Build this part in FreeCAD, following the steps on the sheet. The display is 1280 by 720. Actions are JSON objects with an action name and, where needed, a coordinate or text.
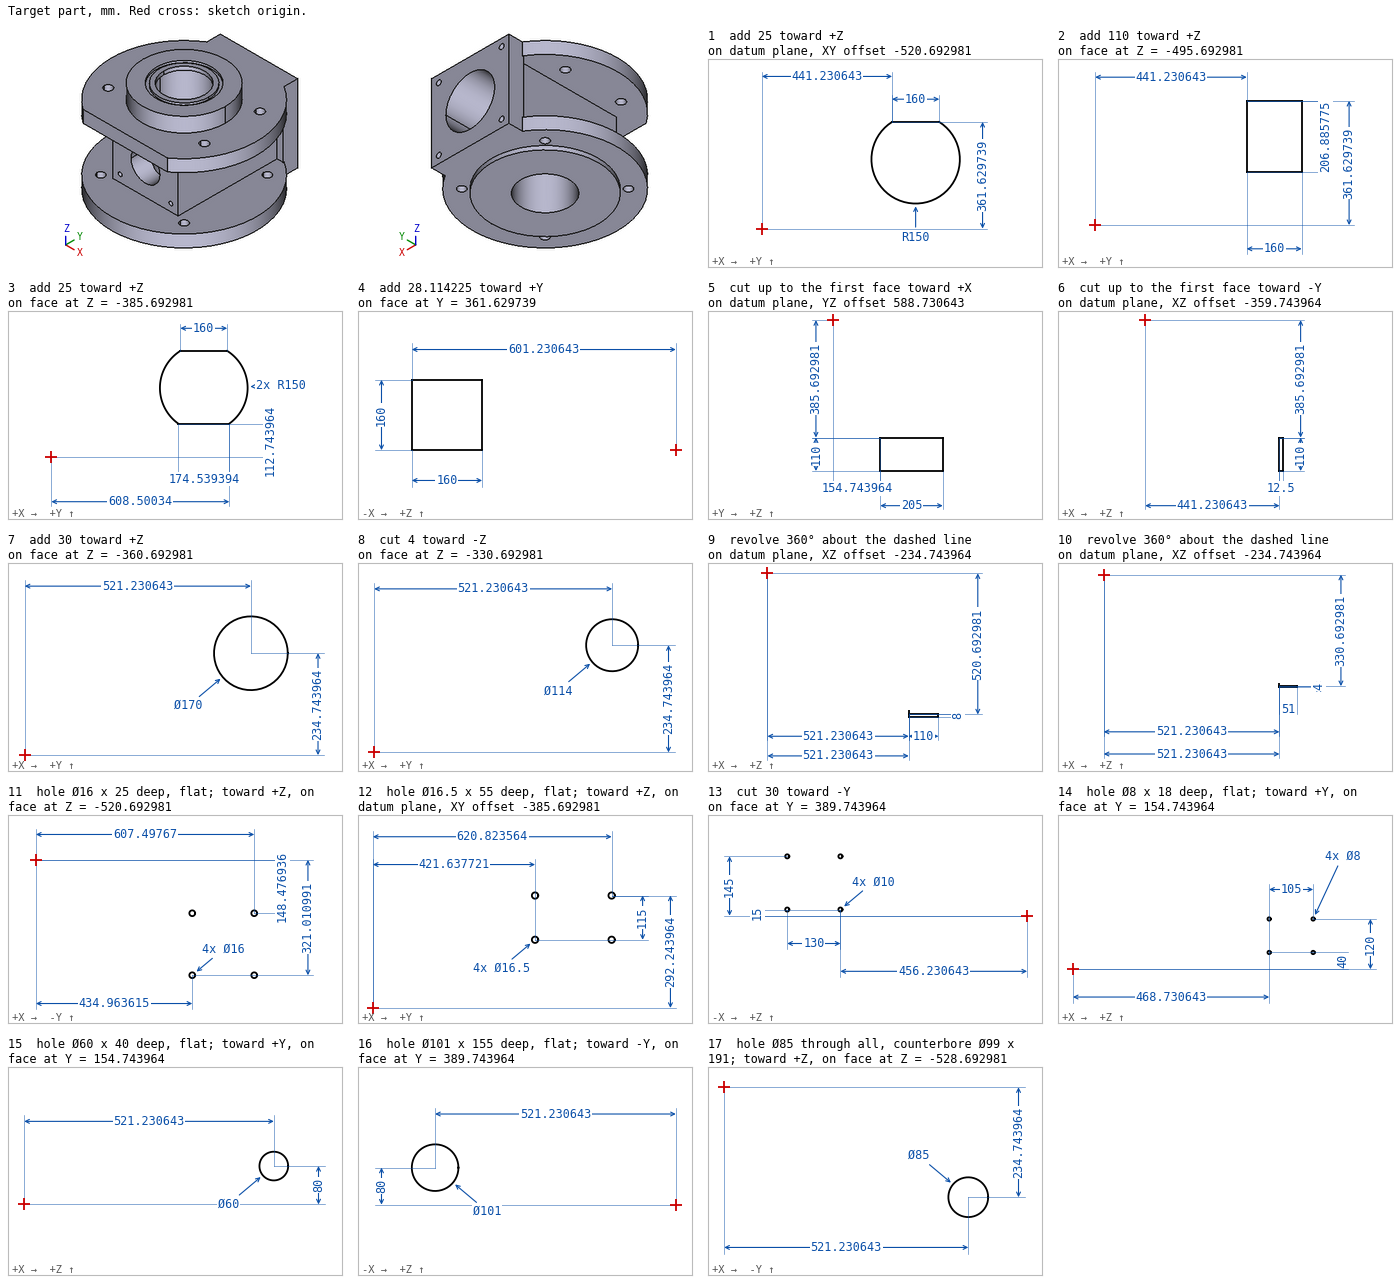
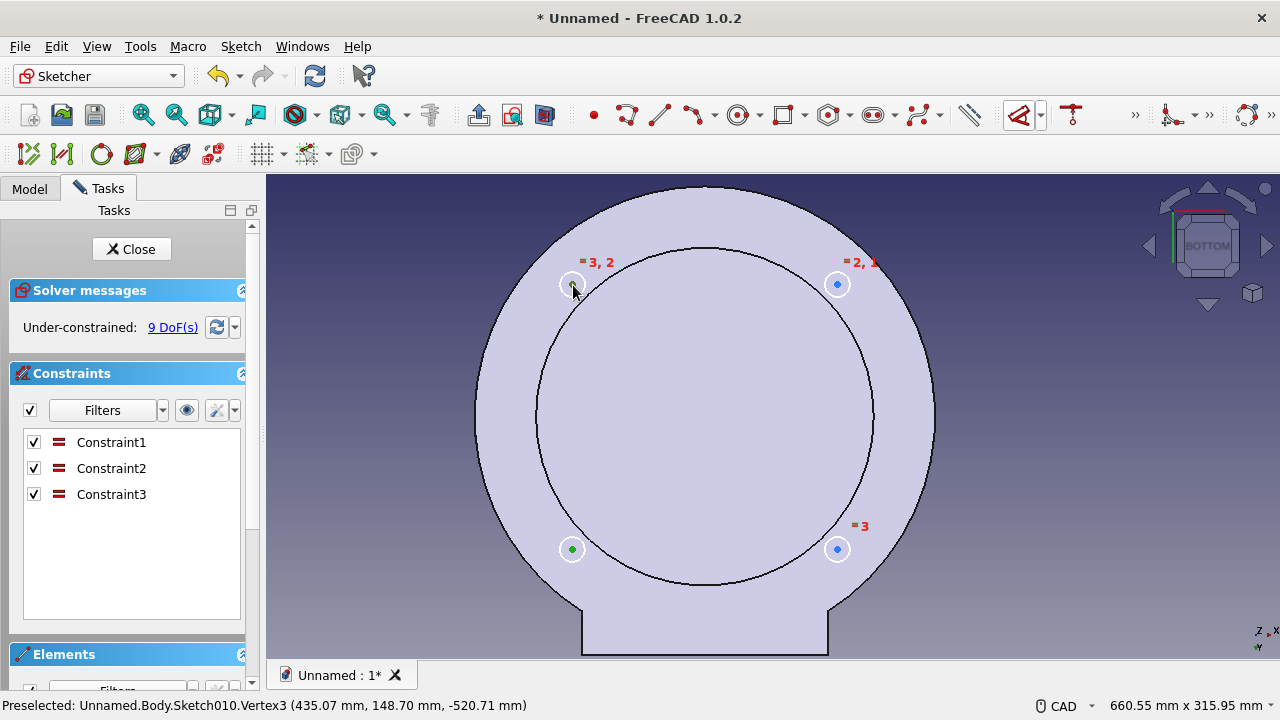
{"action": "key", "text": "v"}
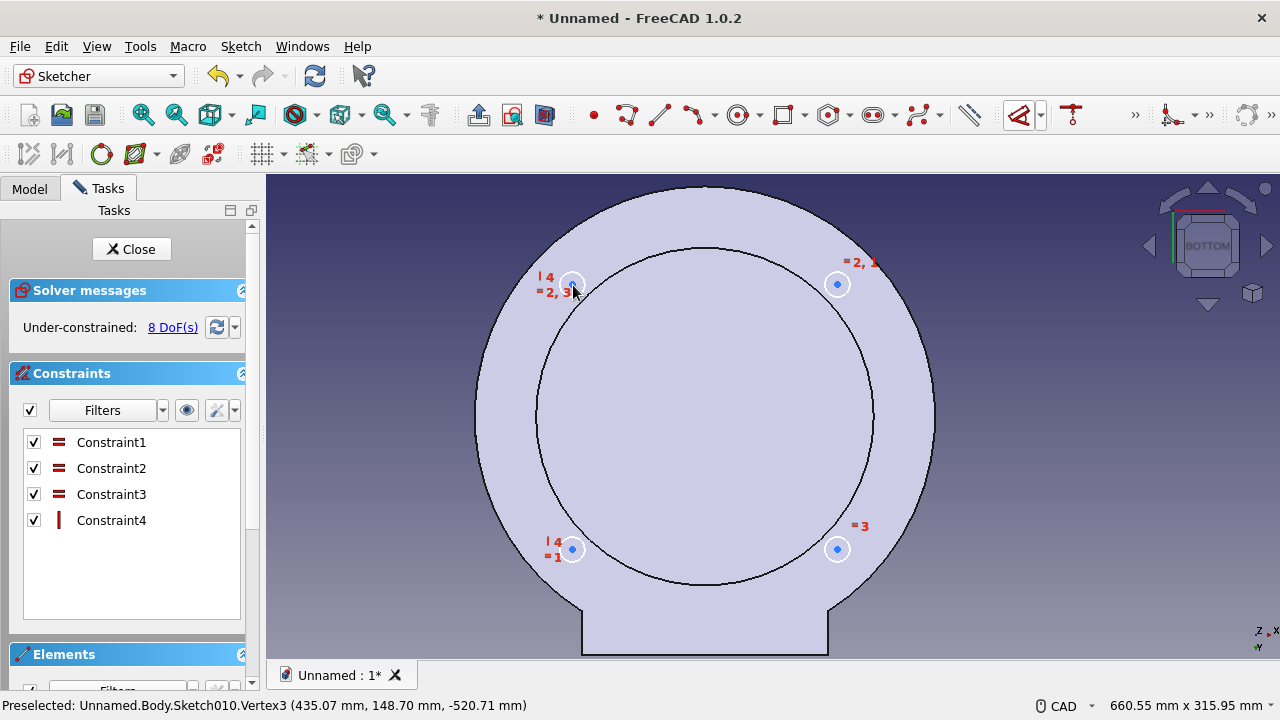
{"action": "left_click", "coordinate": [837, 285]}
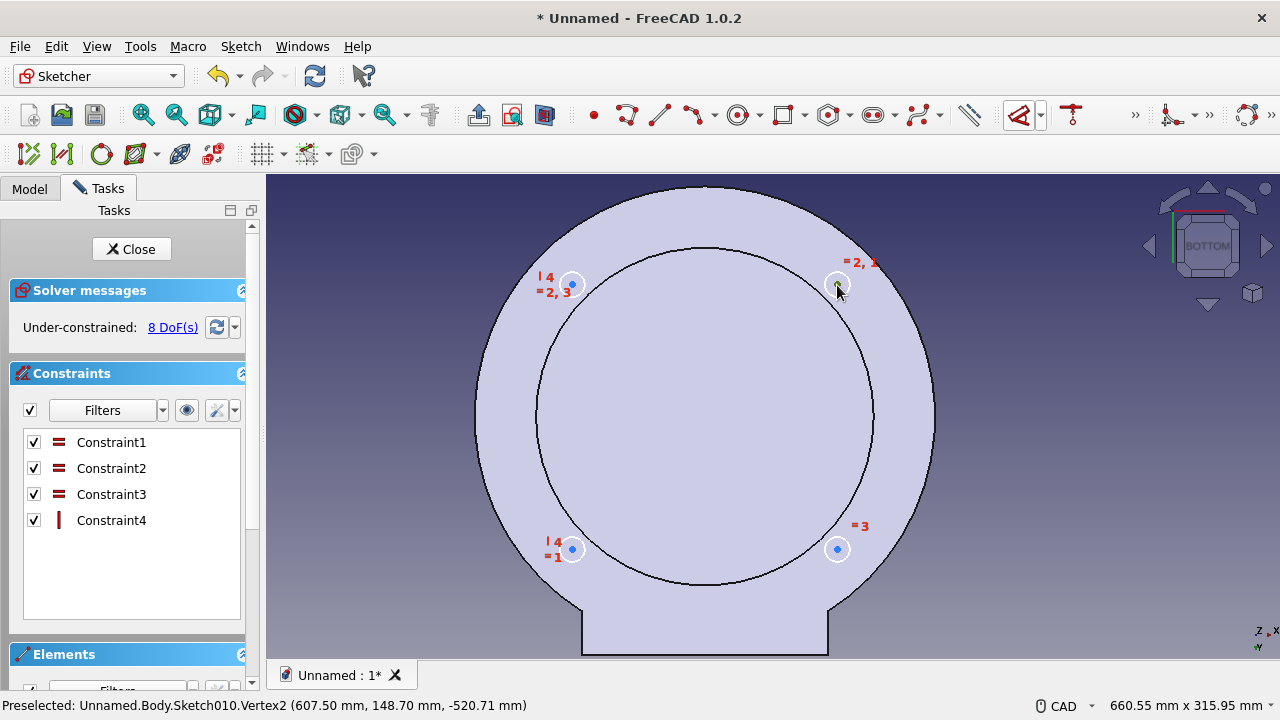
{"action": "left_click", "coordinate": [572, 285]}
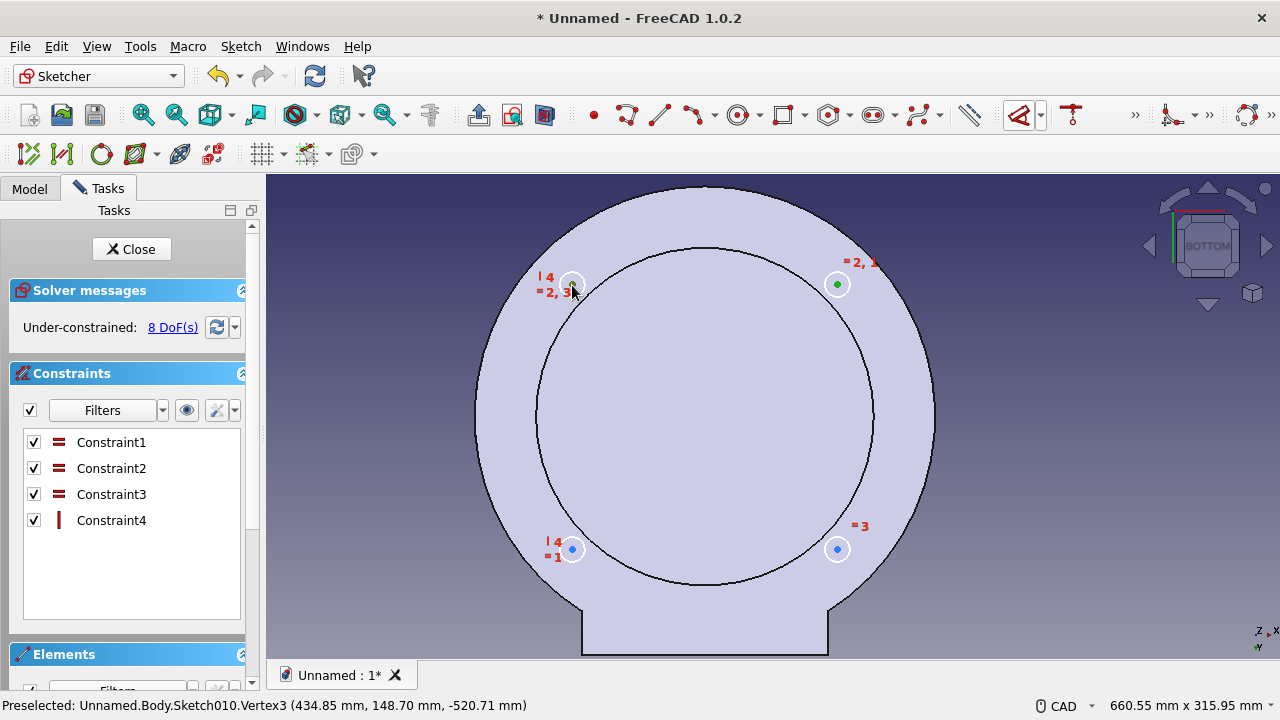
{"action": "key", "text": "h"}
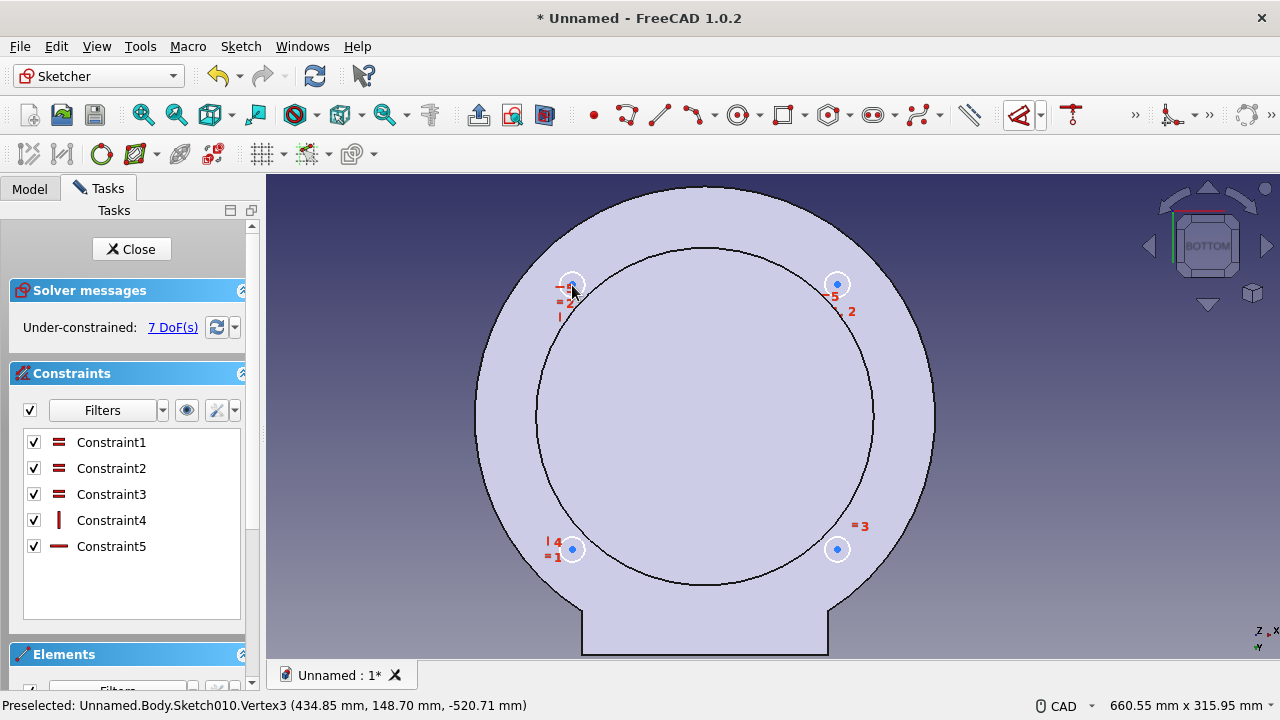
{"action": "left_click", "coordinate": [837, 285]}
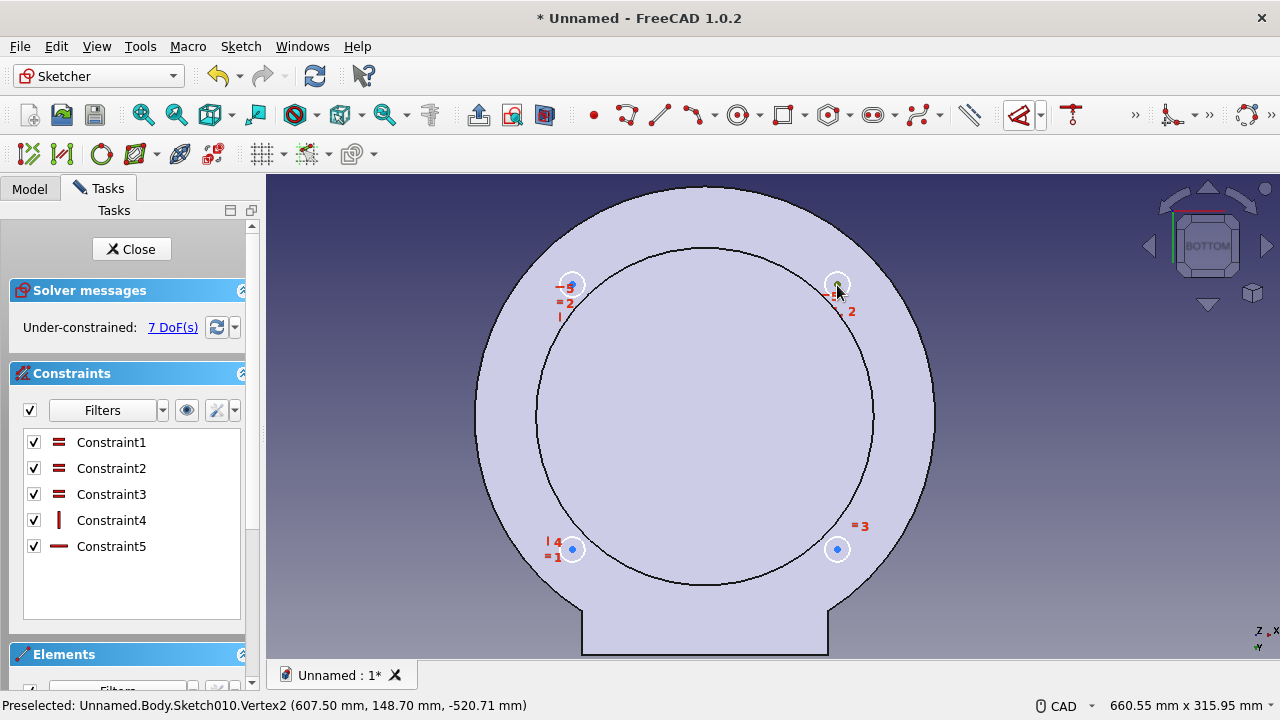
{"action": "left_click", "coordinate": [837, 549]}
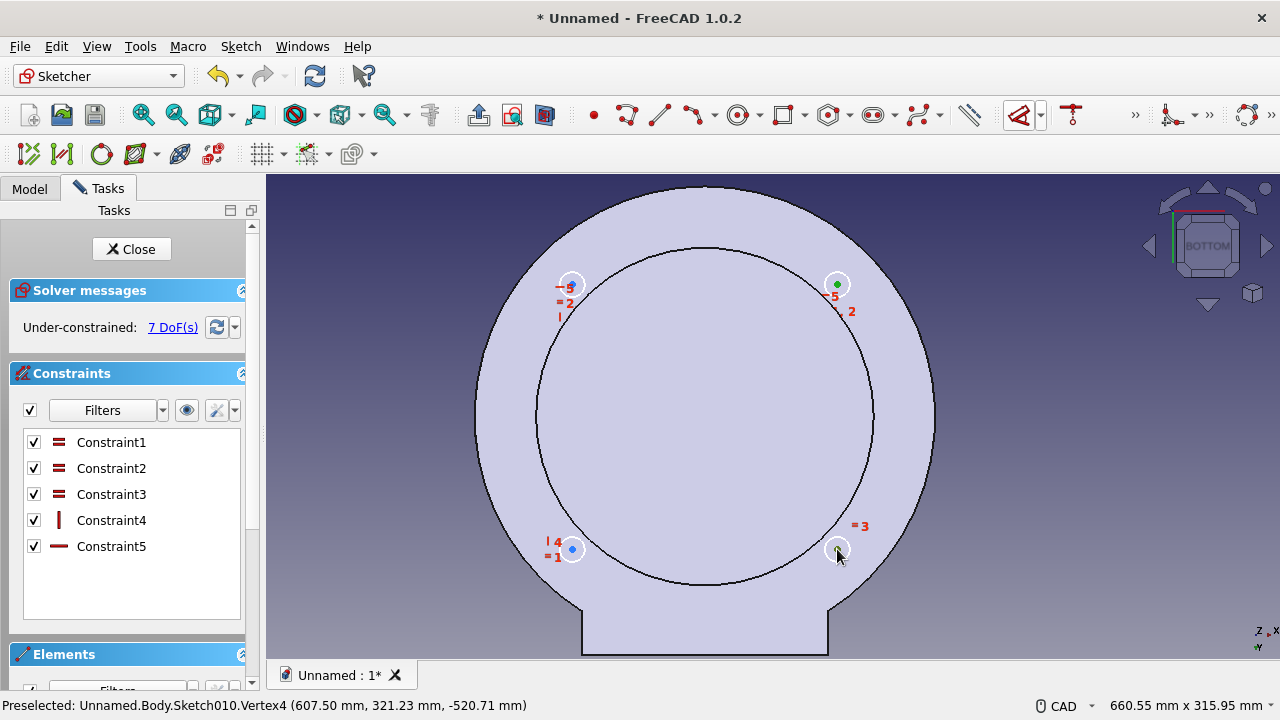
{"action": "key", "text": "v"}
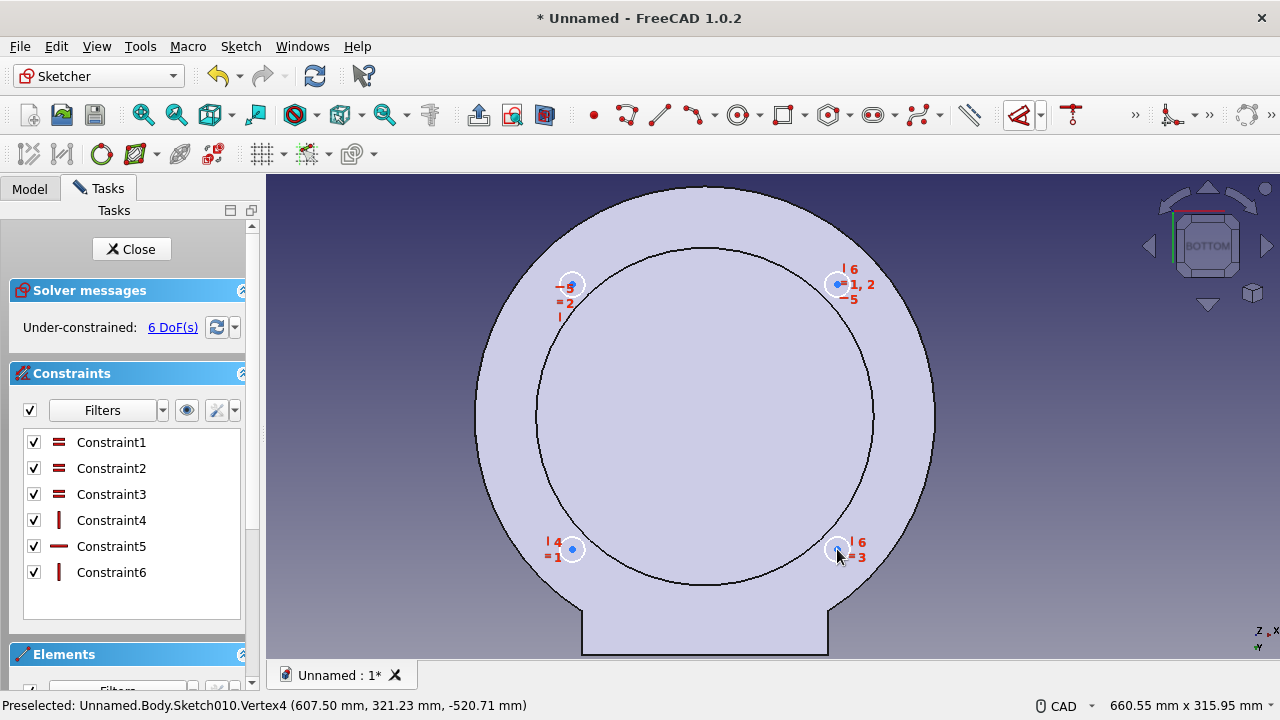
{"action": "left_click", "coordinate": [572, 550]}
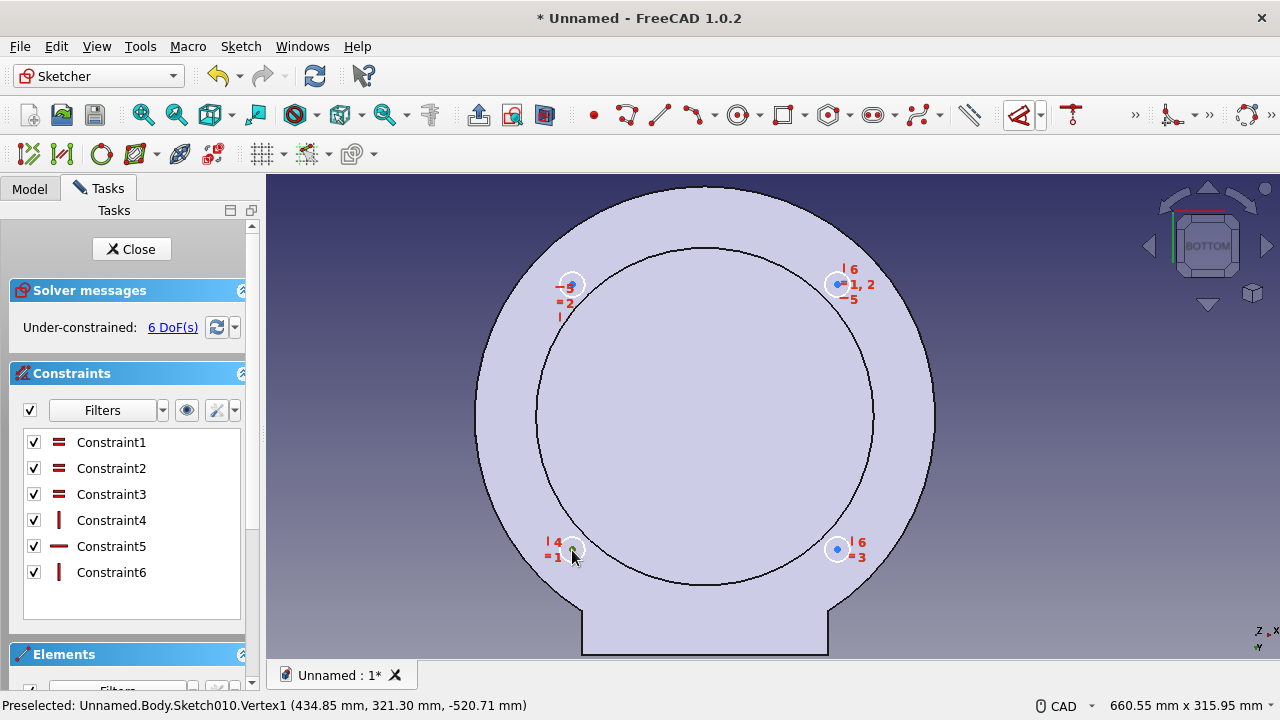
{"action": "left_click", "coordinate": [837, 549]}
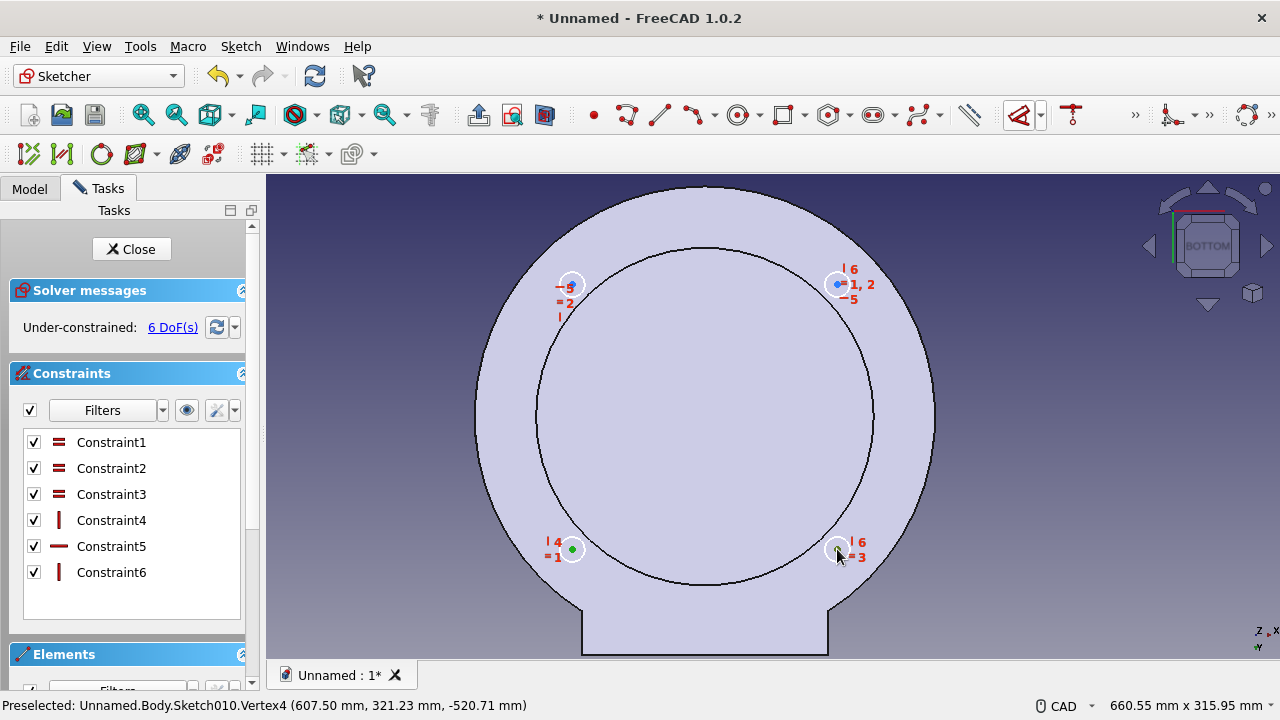
{"action": "key", "text": "h"}